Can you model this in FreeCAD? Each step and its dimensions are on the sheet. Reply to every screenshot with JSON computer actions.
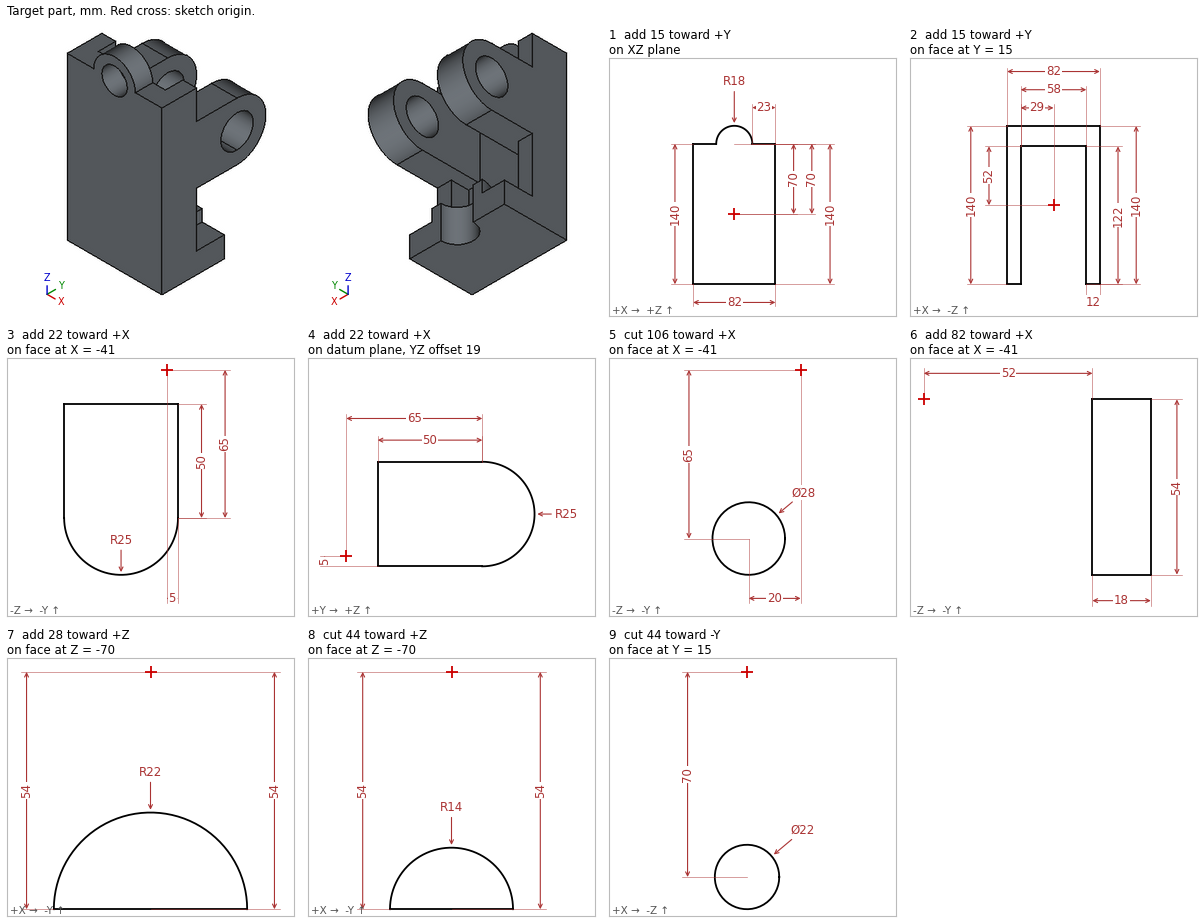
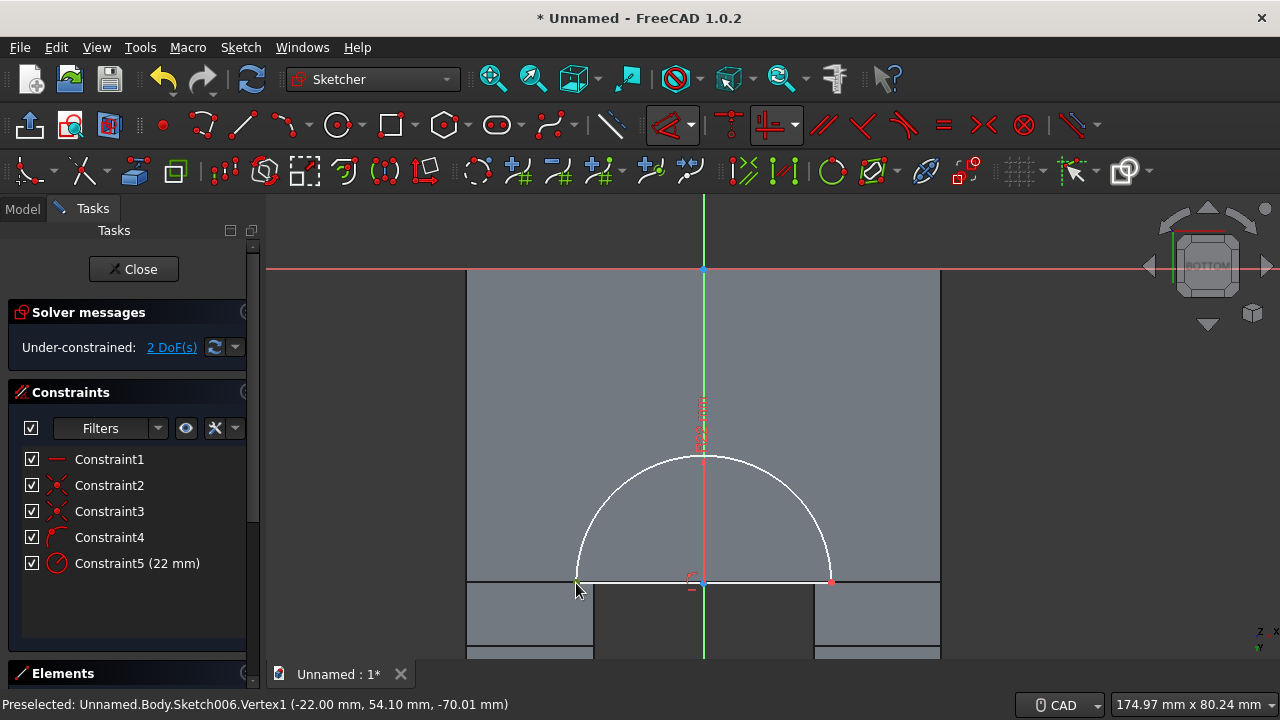
{"action": "key", "text": "i"}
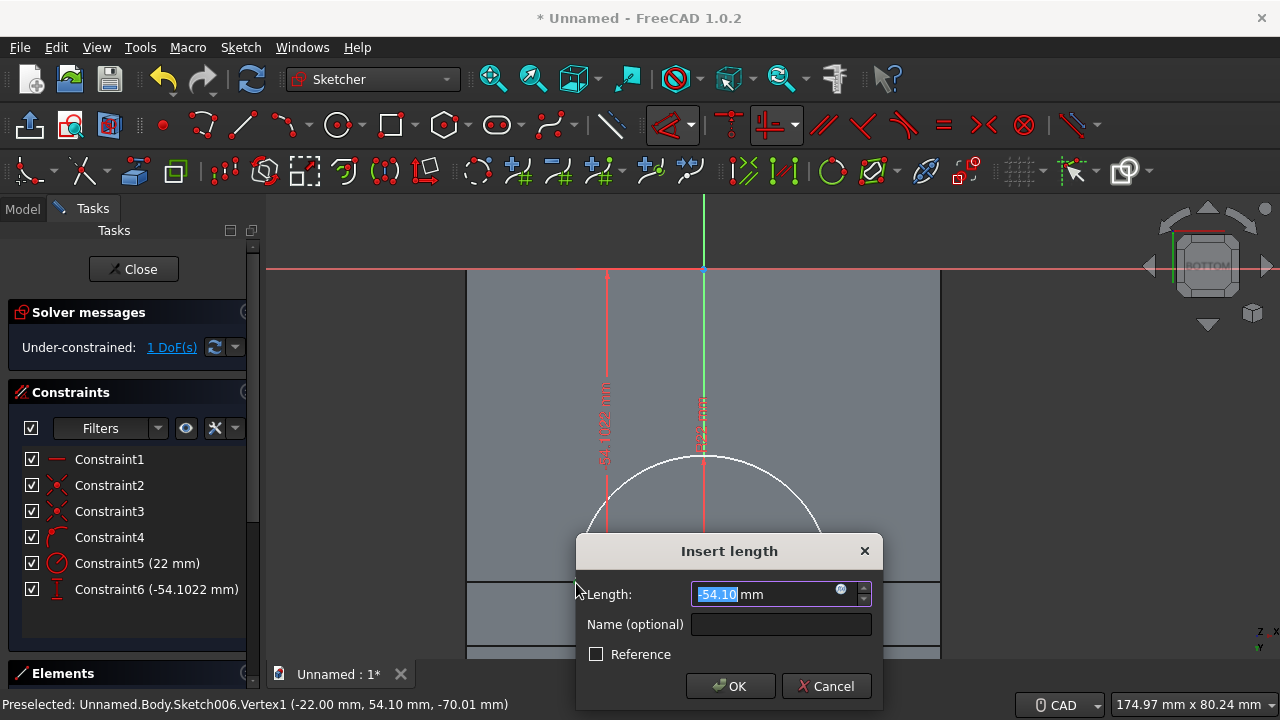
{"action": "type", "text": "-54"}
{"action": "key", "text": "Return"}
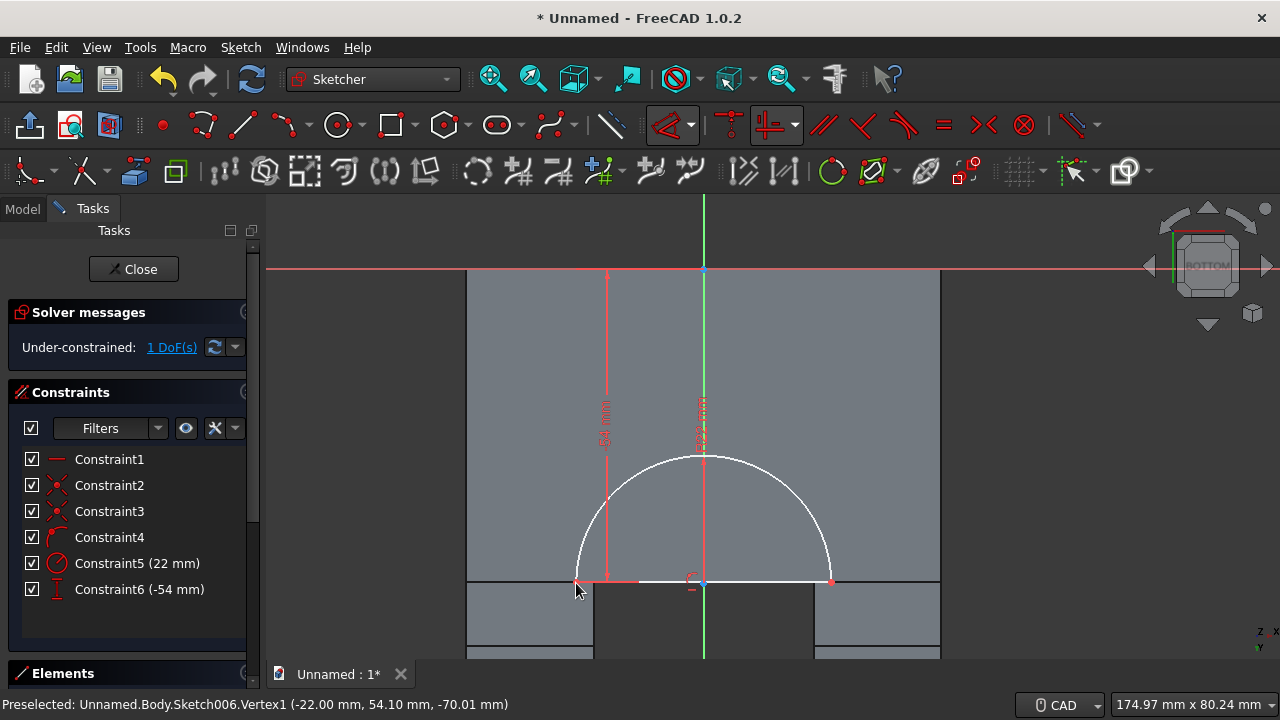
{"action": "left_click", "coordinate": [704, 583]}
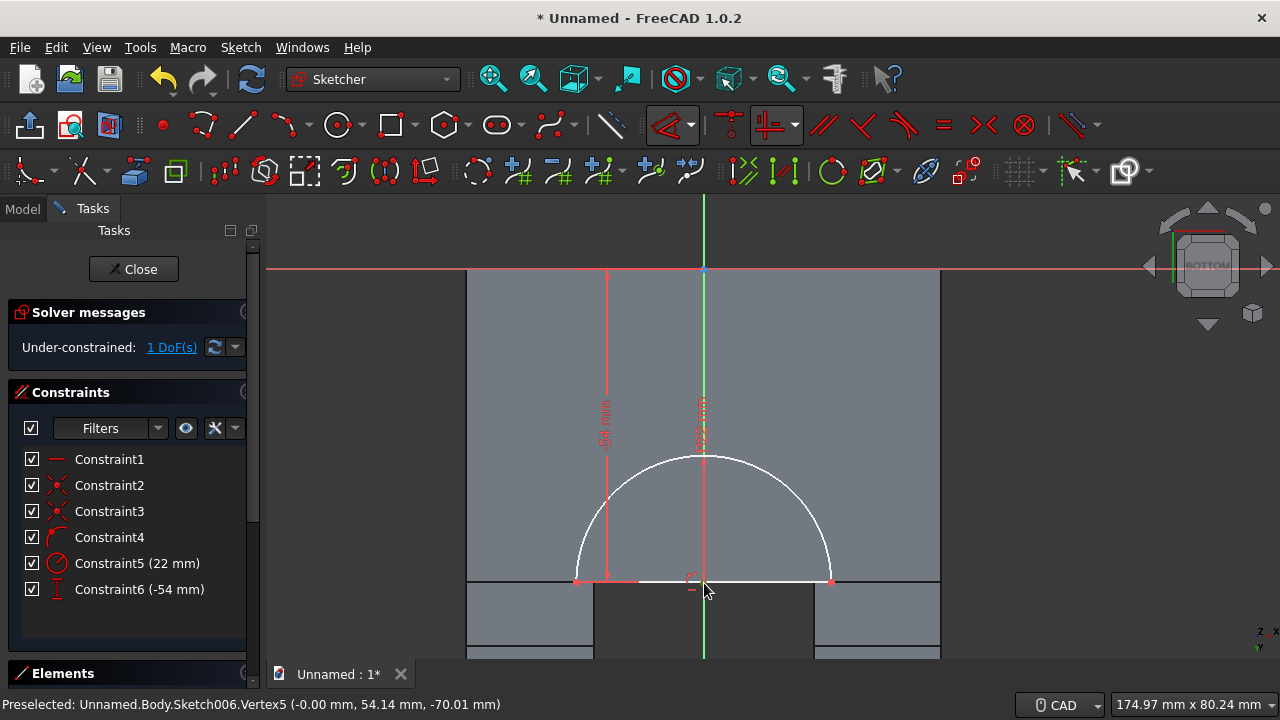
{"action": "key", "text": "i"}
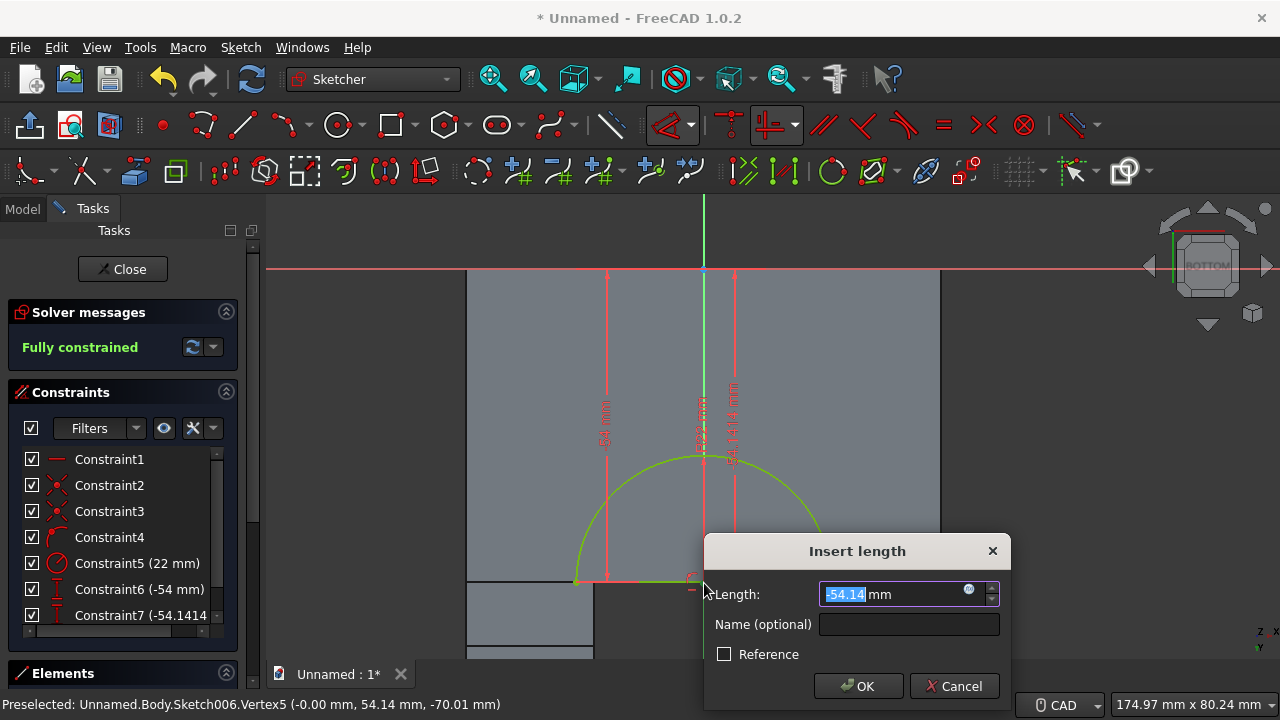
{"action": "type", "text": "-54"}
{"action": "key", "text": "Return"}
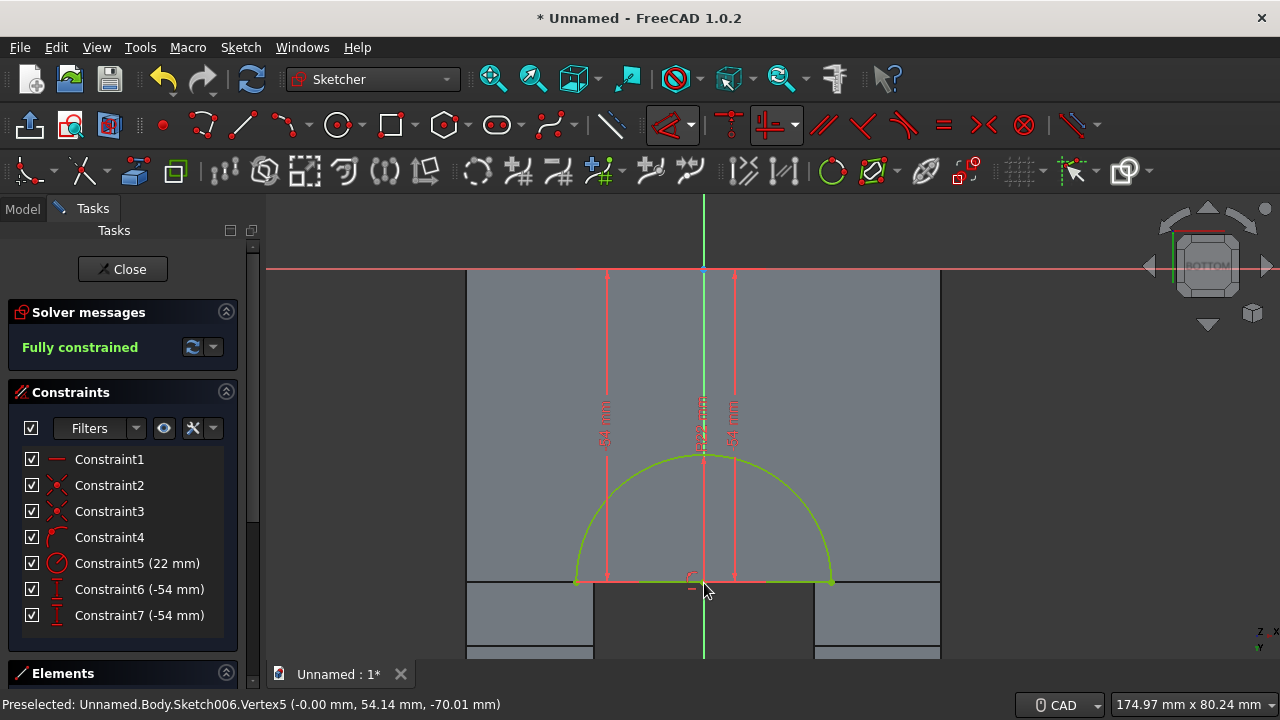
{"action": "left_click", "coordinate": [123, 269]}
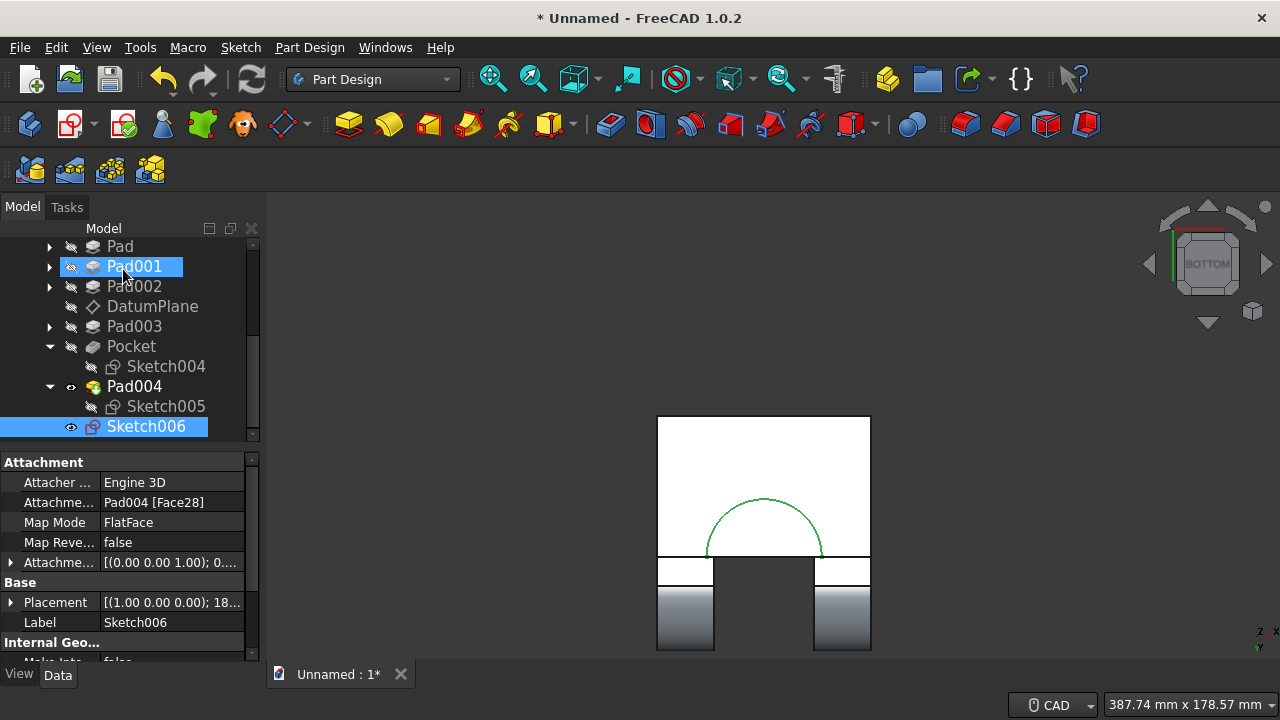
{"action": "left_click", "coordinate": [350, 124]}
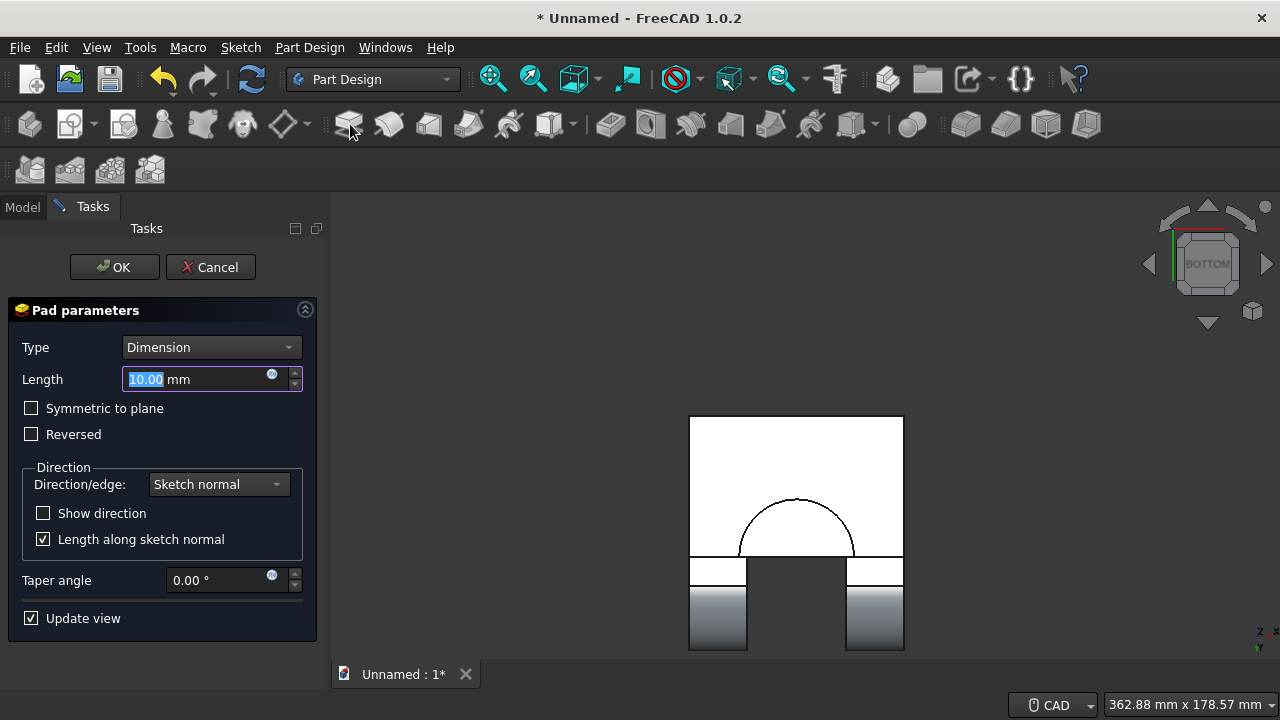
{"action": "type", "text": "28"}
{"action": "key", "text": "Tab"}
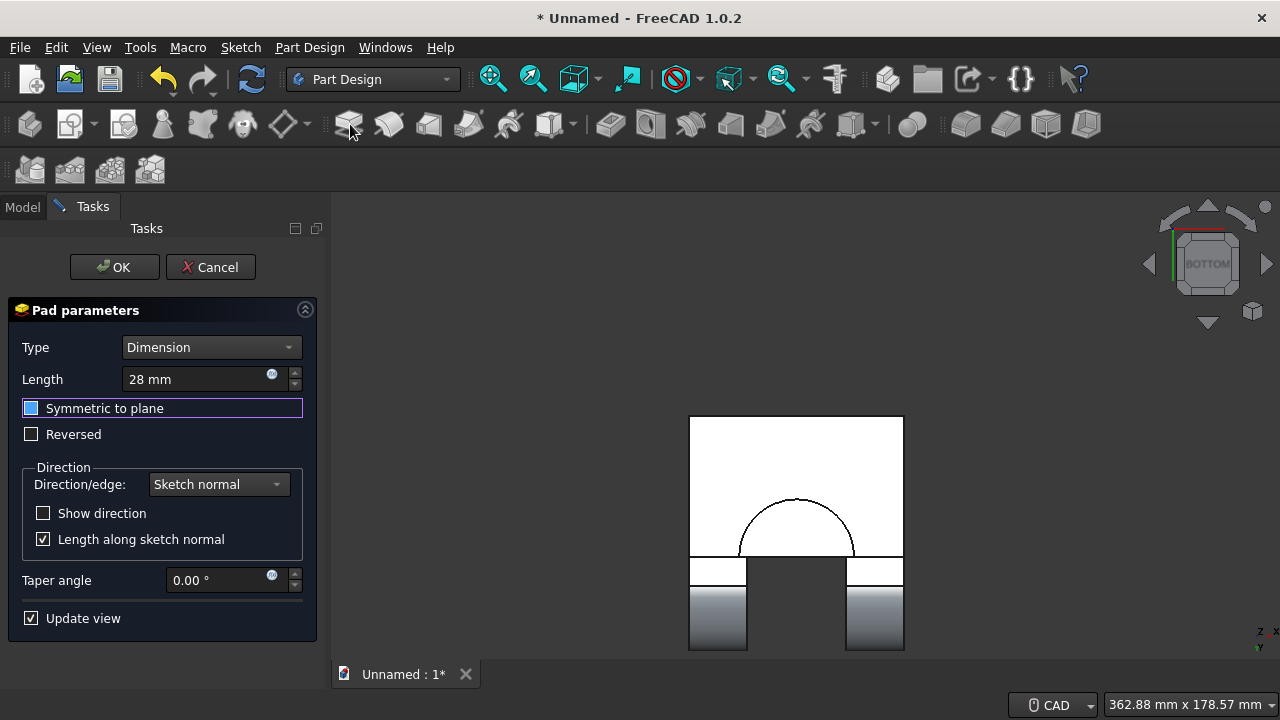
{"action": "left_click", "coordinate": [30, 434]}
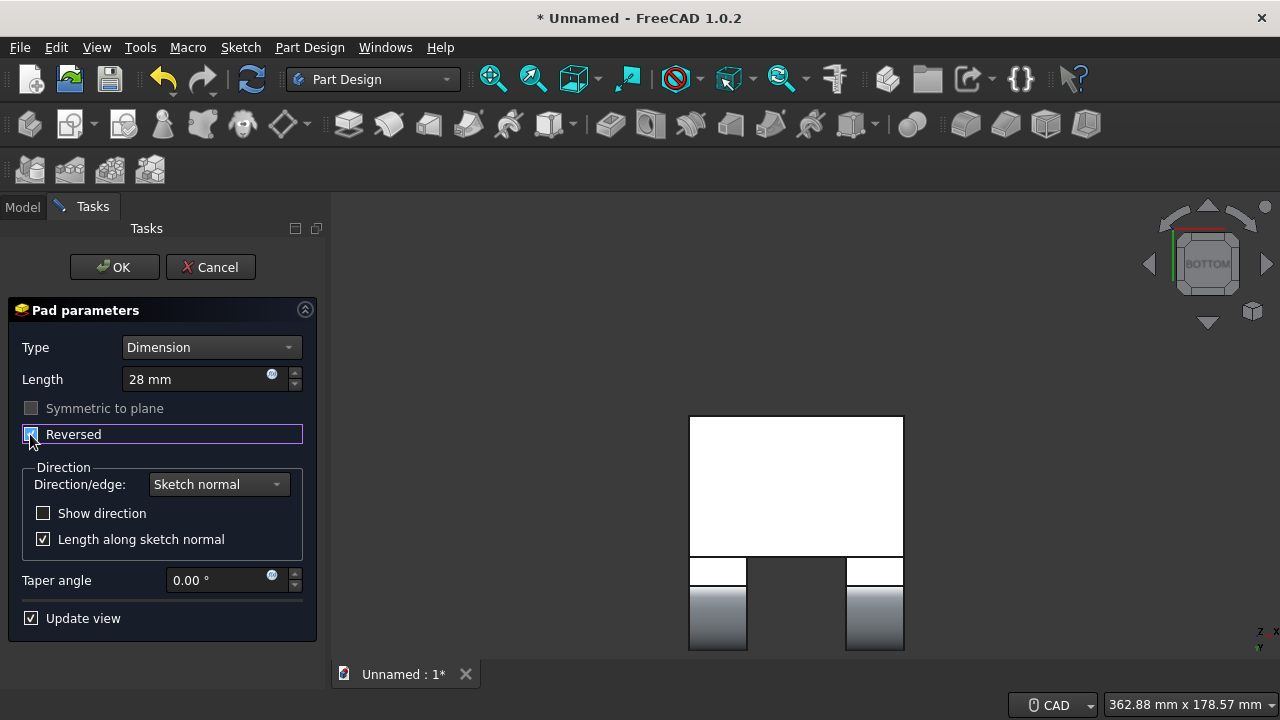
{"action": "left_click", "coordinate": [115, 267]}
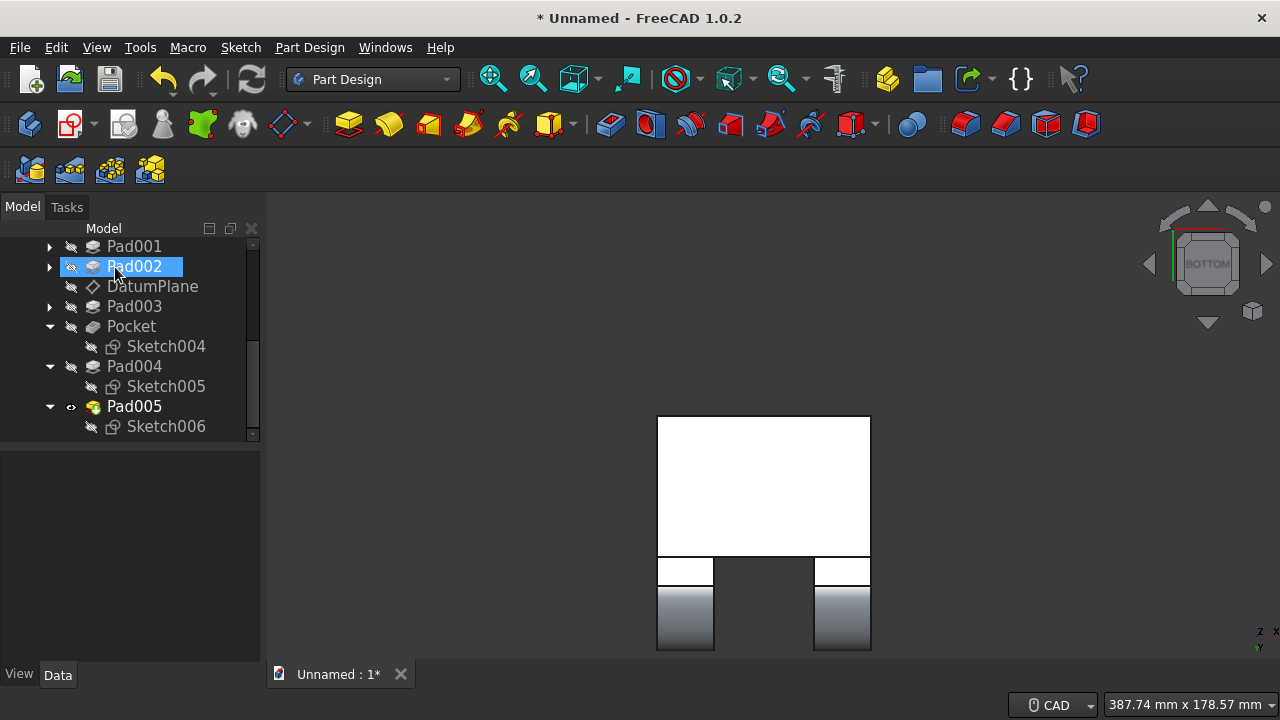
{"action": "left_click", "coordinate": [795, 485]}